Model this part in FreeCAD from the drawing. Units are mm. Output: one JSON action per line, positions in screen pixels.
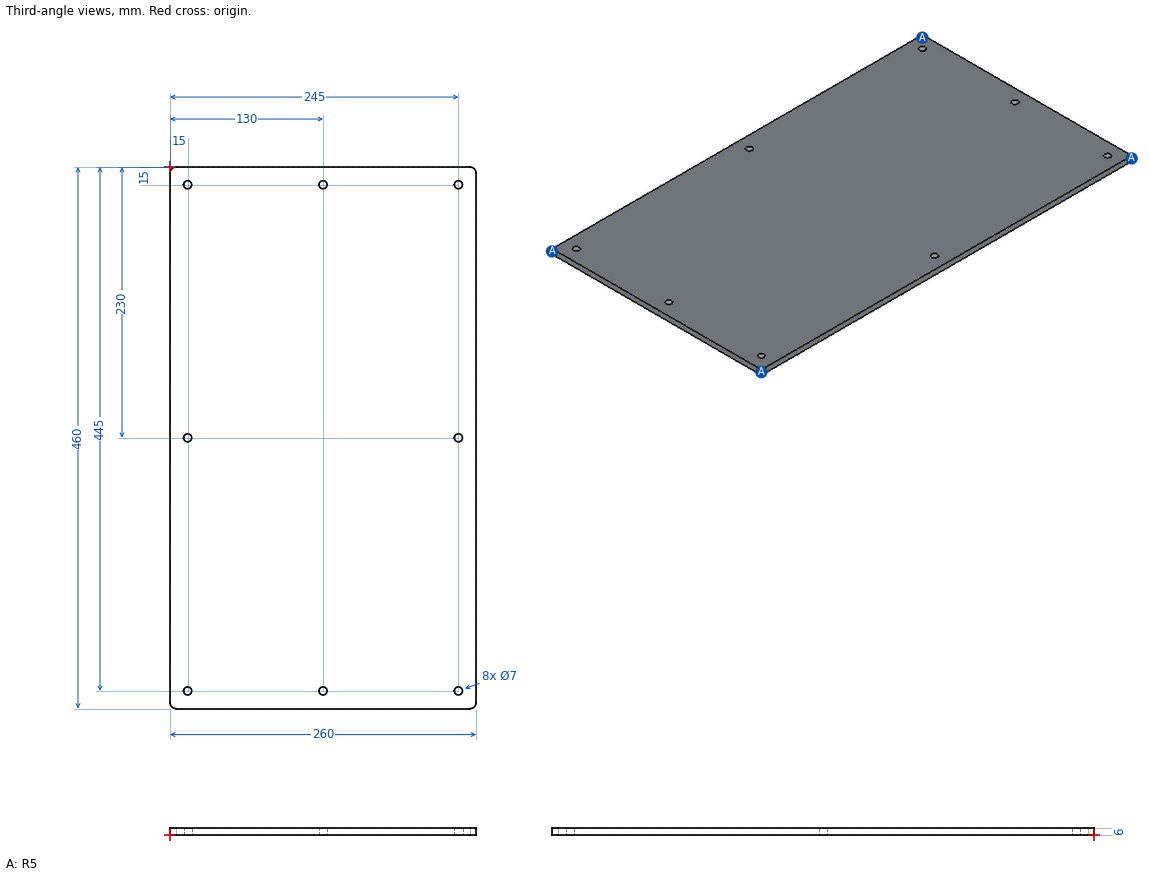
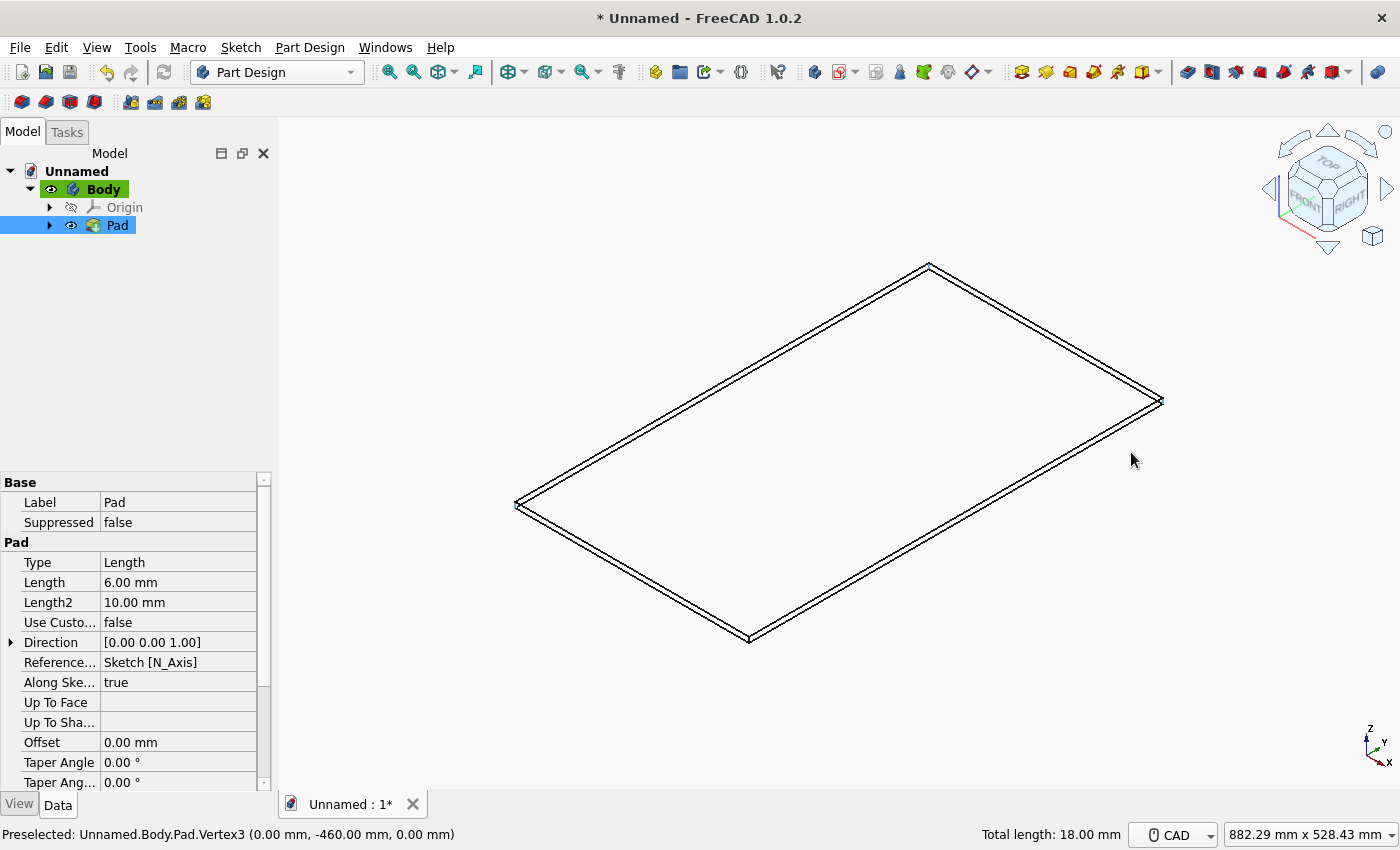
{"action": "scroll", "coordinate": [749, 639], "scroll_direction": "up", "scroll_amount": 9}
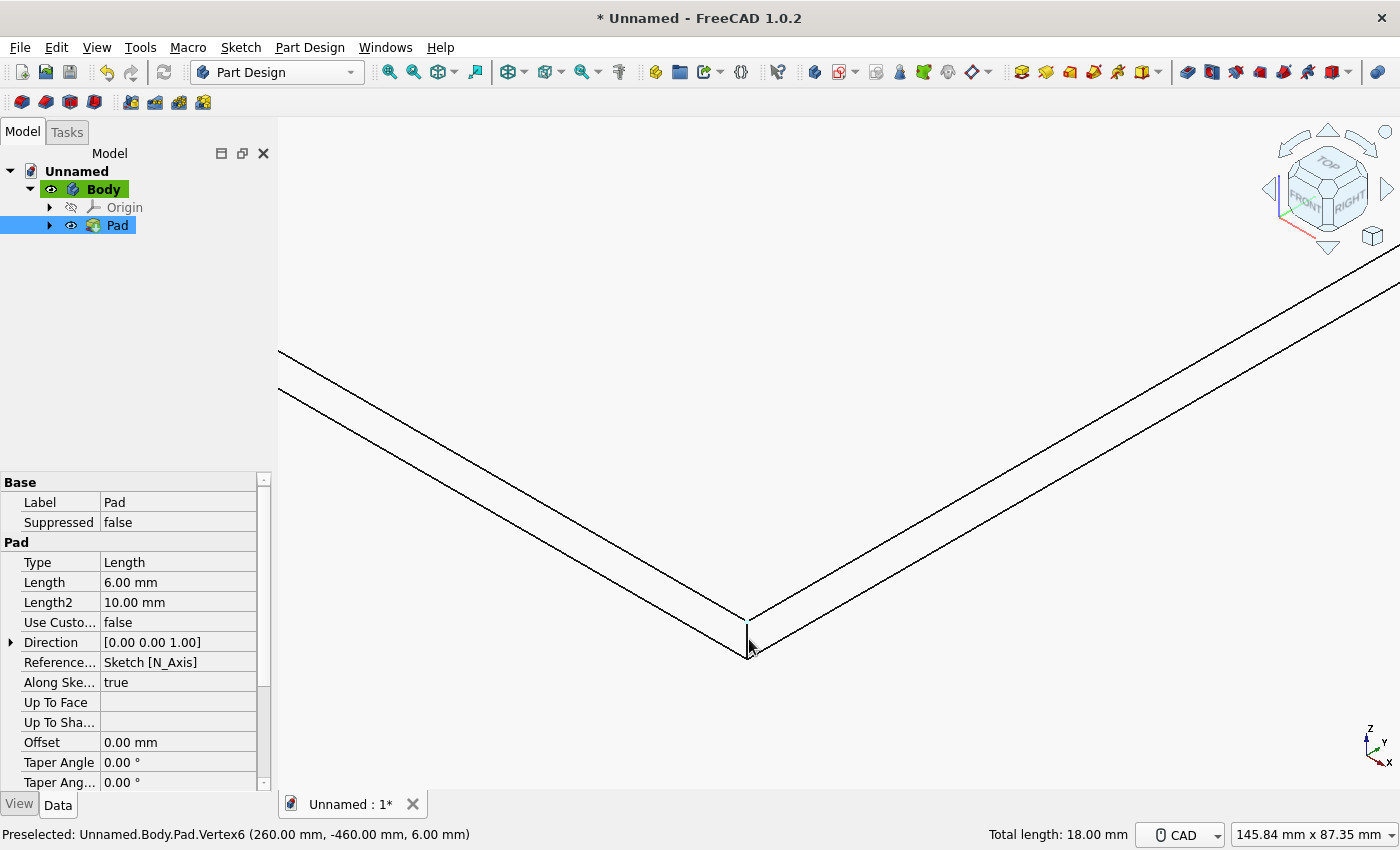
{"action": "left_click", "coordinate": [747, 640], "text": "ctrl"}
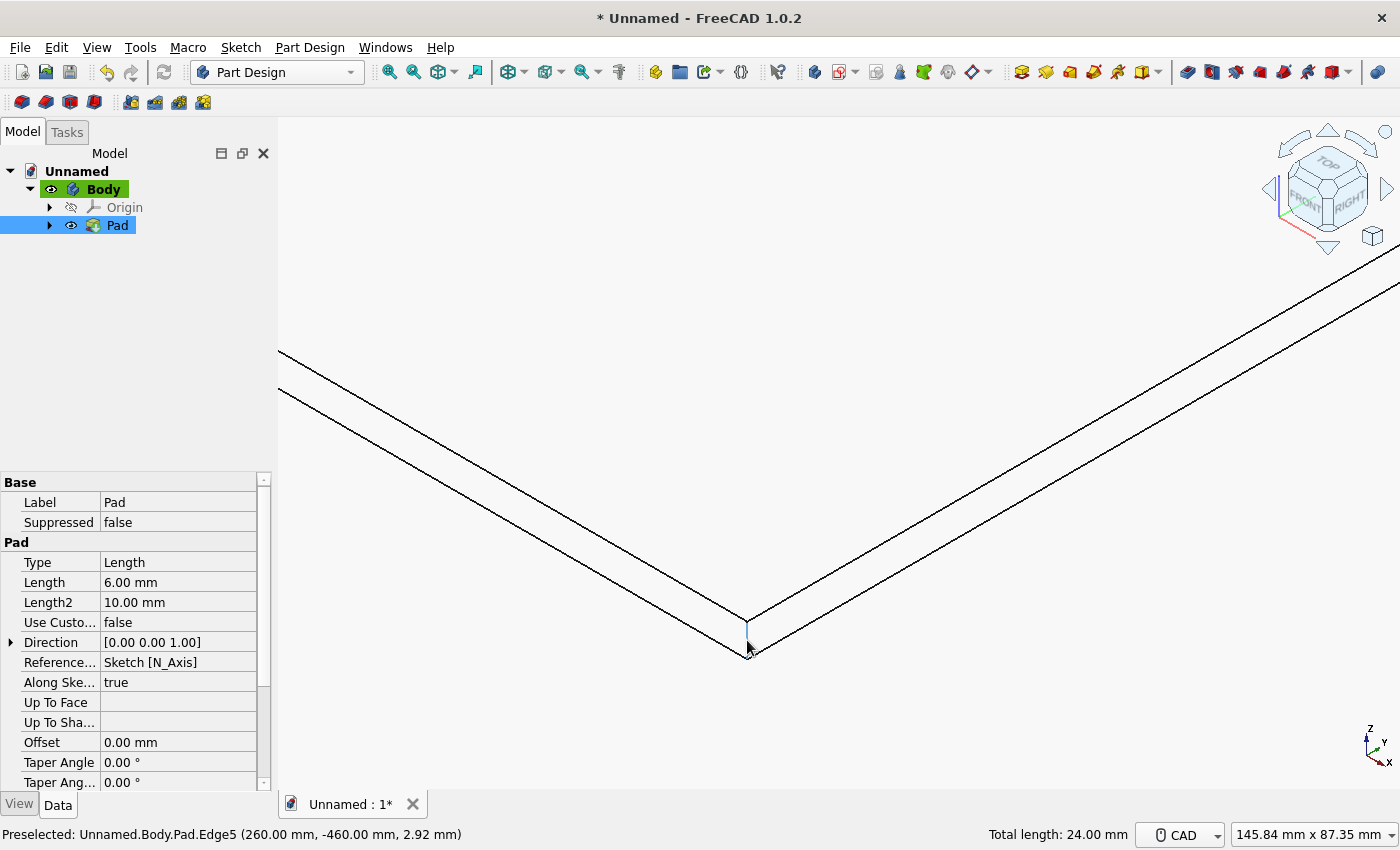
{"action": "key", "text": "v 1"}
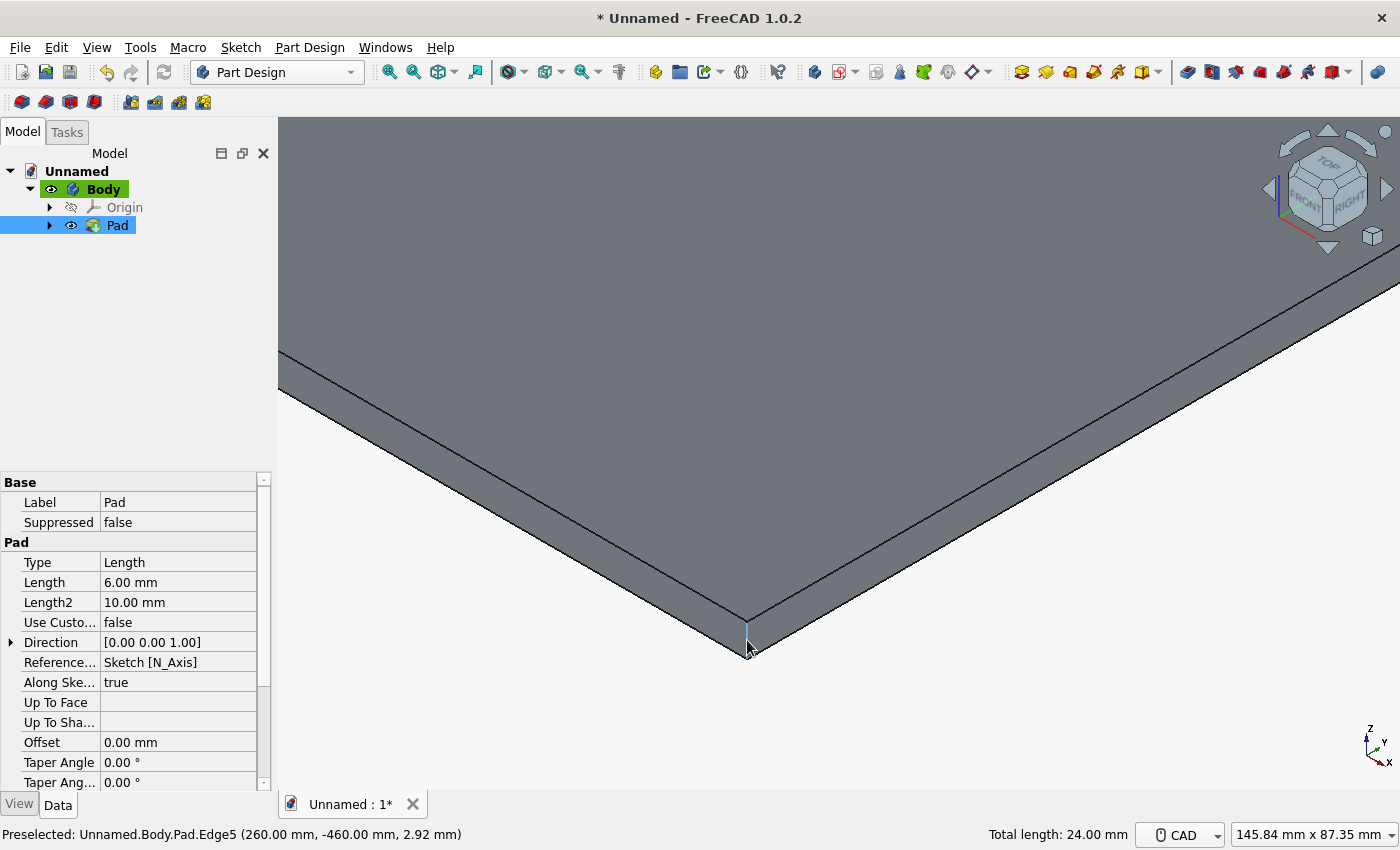
{"action": "left_click", "coordinate": [22, 102]}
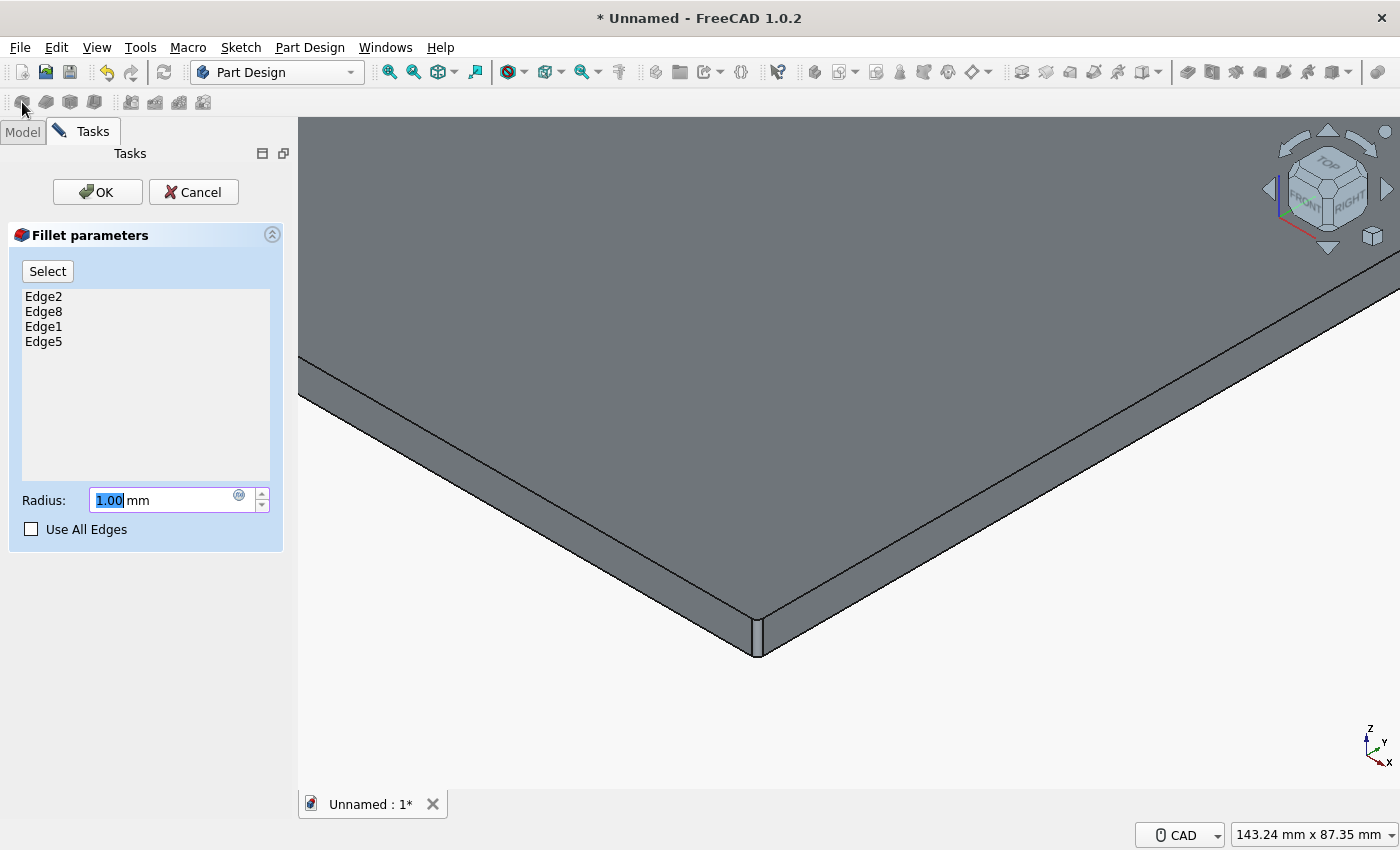
{"action": "type", "text": "5"}
{"action": "key", "text": "Tab"}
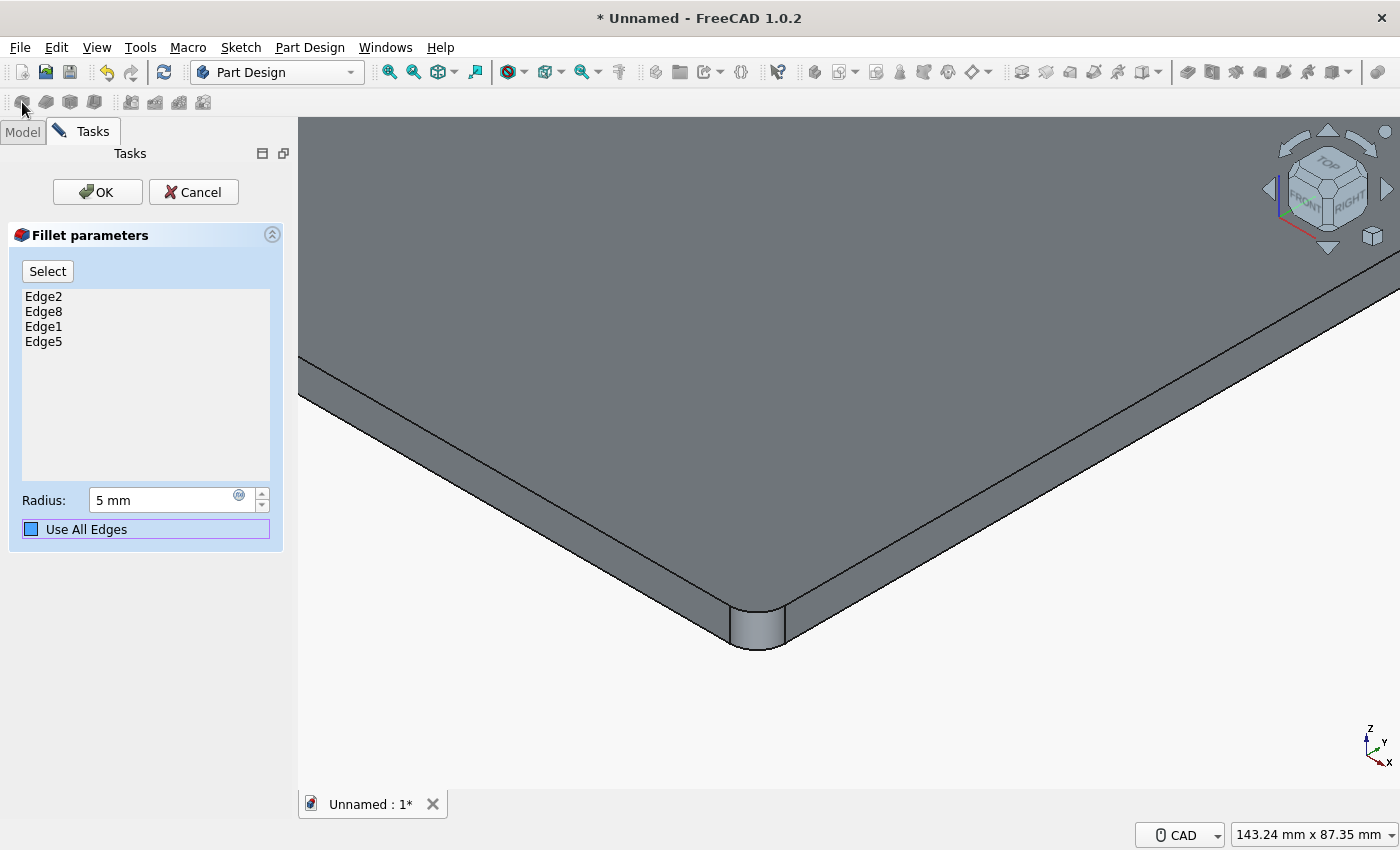
{"action": "left_click", "coordinate": [98, 192]}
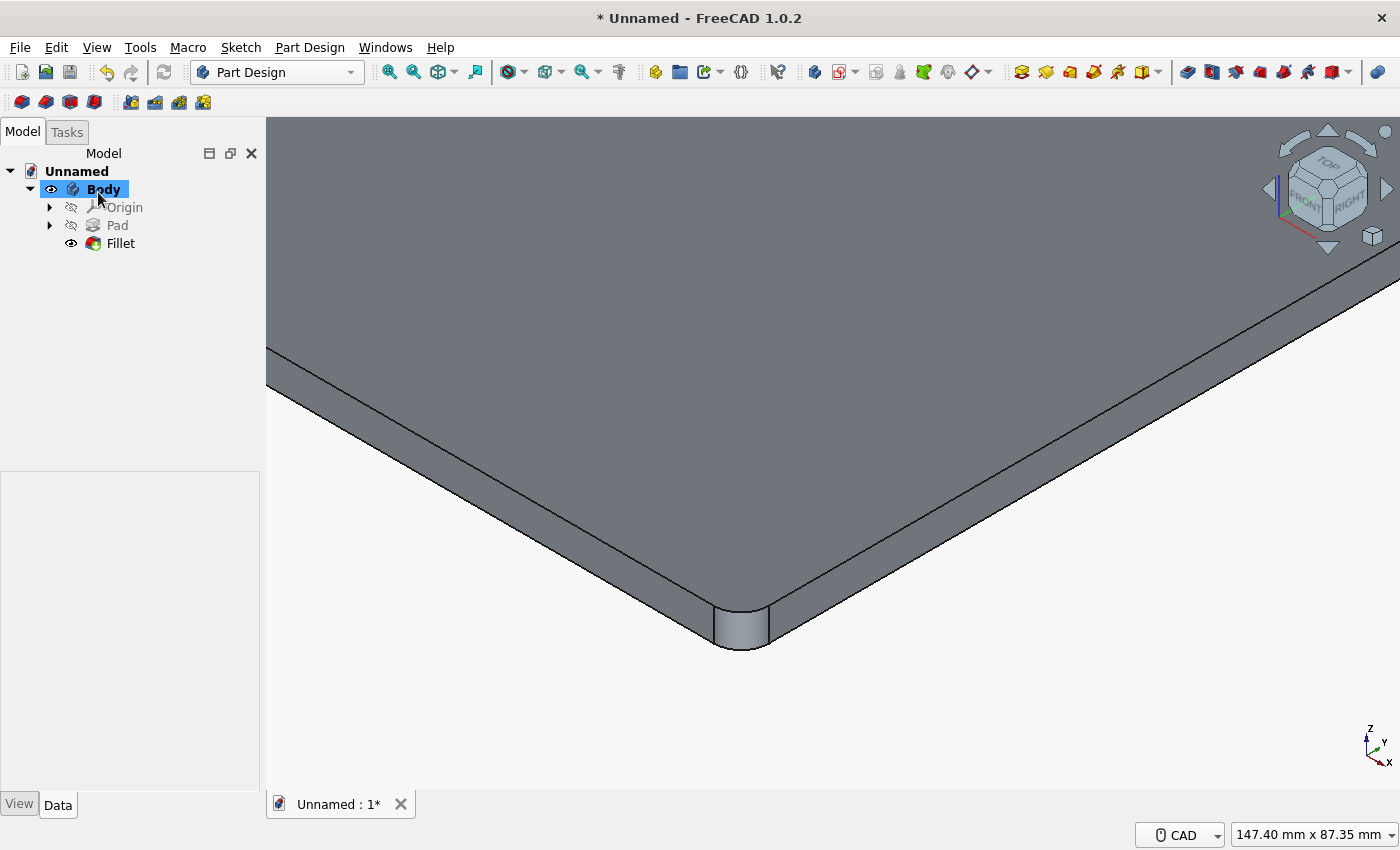
{"action": "key", "text": "v f"}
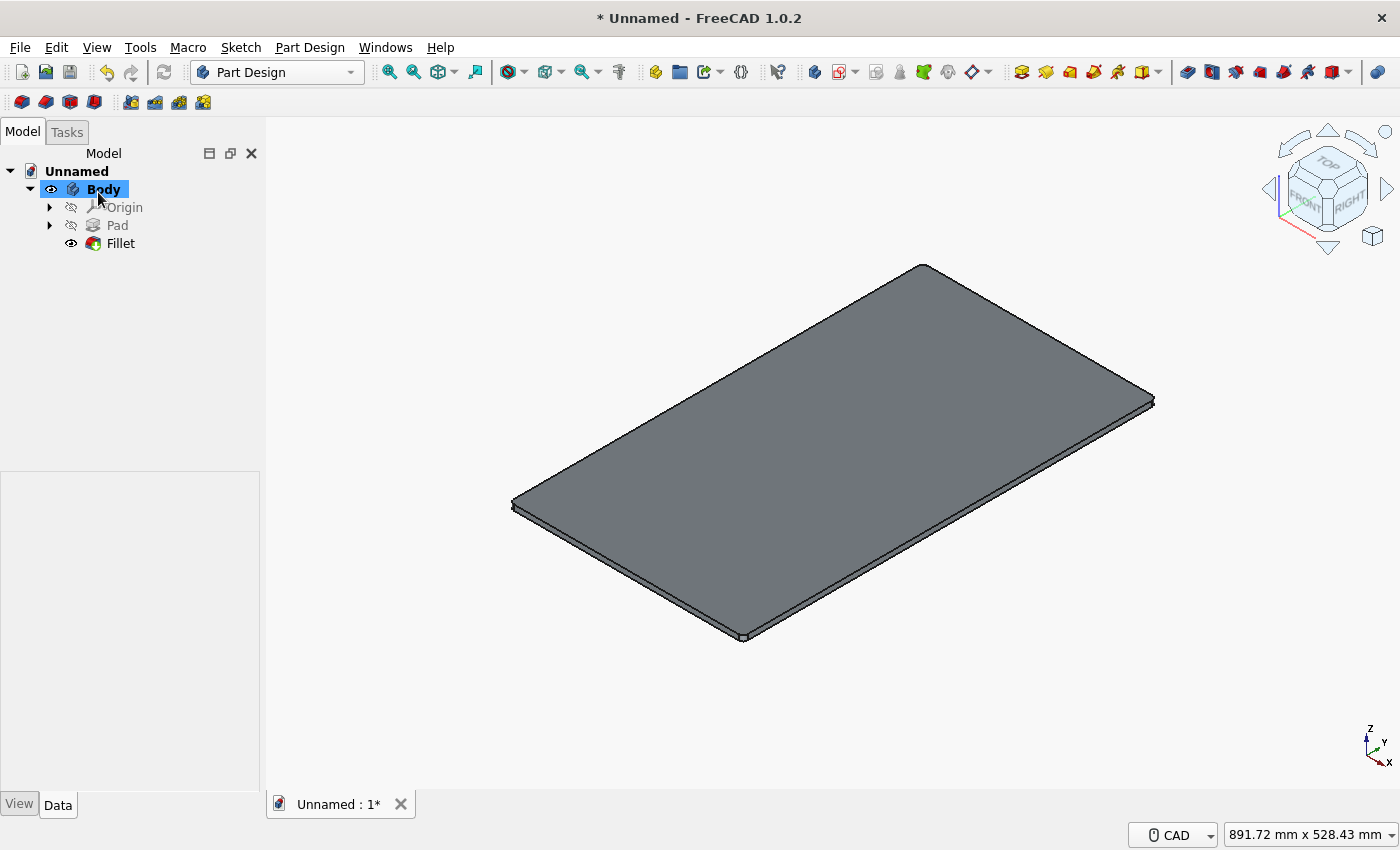
{"action": "left_click", "coordinate": [840, 72]}